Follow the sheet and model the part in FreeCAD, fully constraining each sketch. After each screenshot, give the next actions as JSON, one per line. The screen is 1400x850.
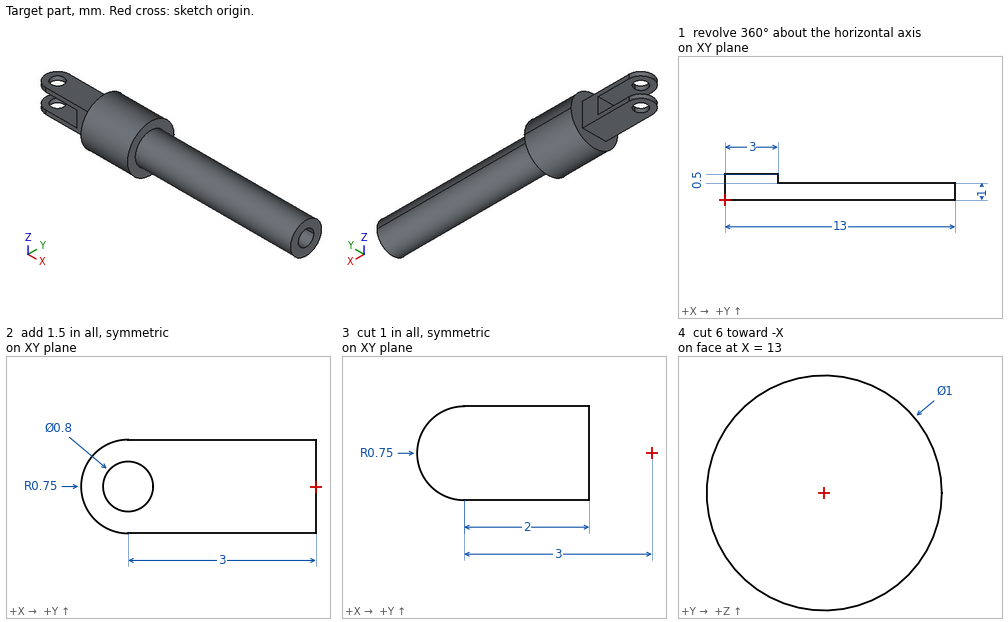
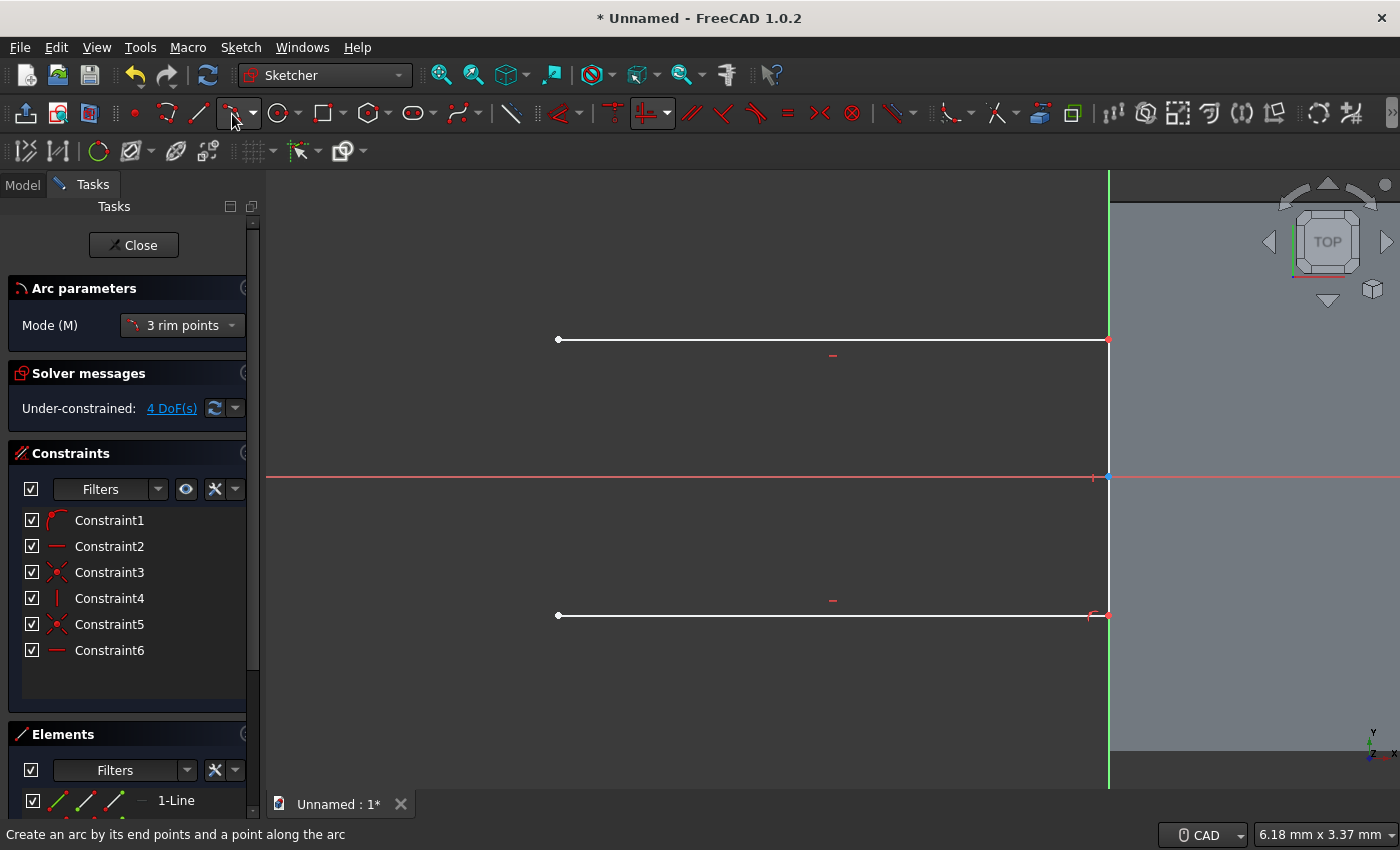
{"action": "left_click", "coordinate": [558, 340]}
{"action": "left_click", "coordinate": [558, 616]}
{"action": "left_click", "coordinate": [427, 434]}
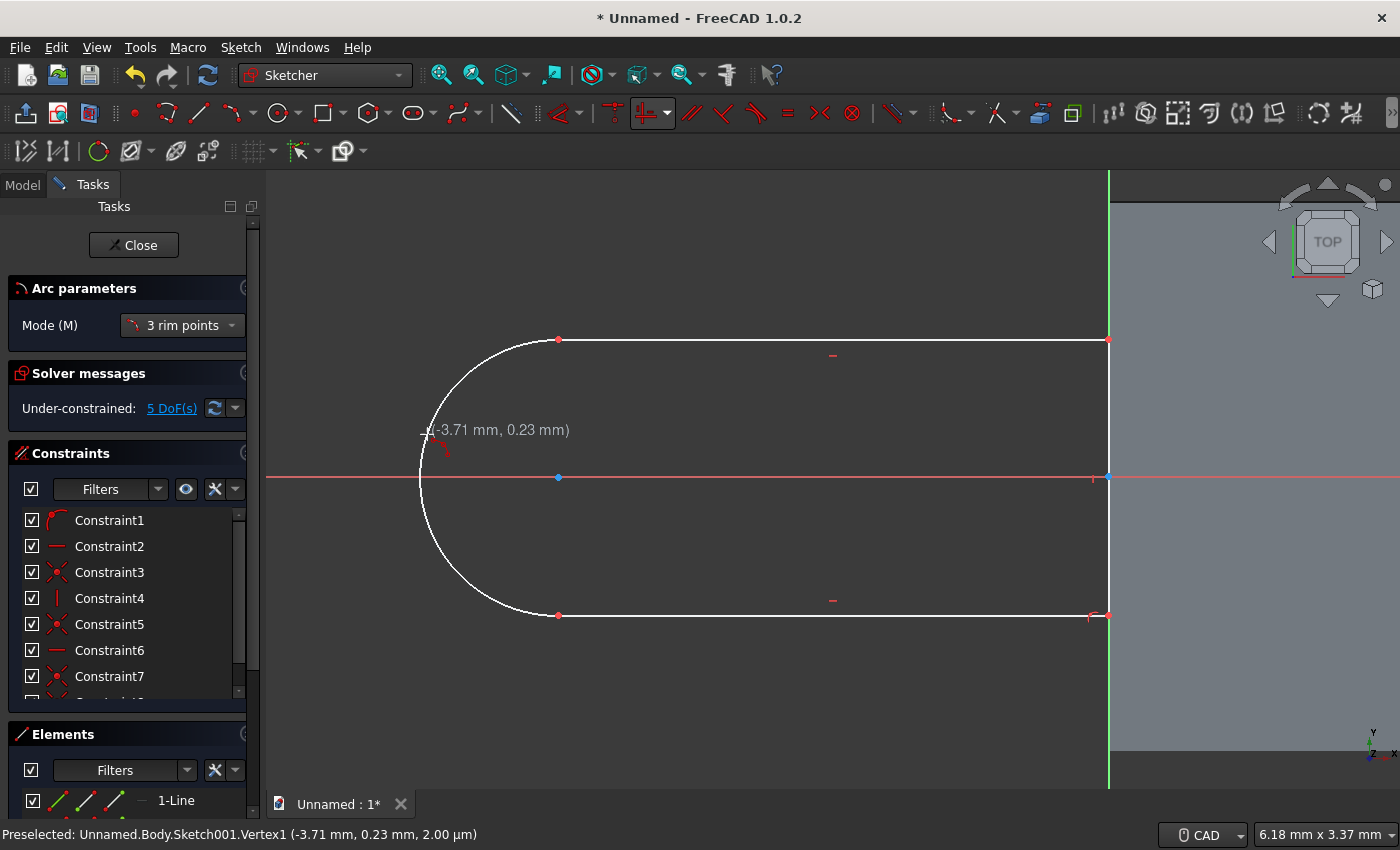
{"action": "left_click", "coordinate": [278, 114]}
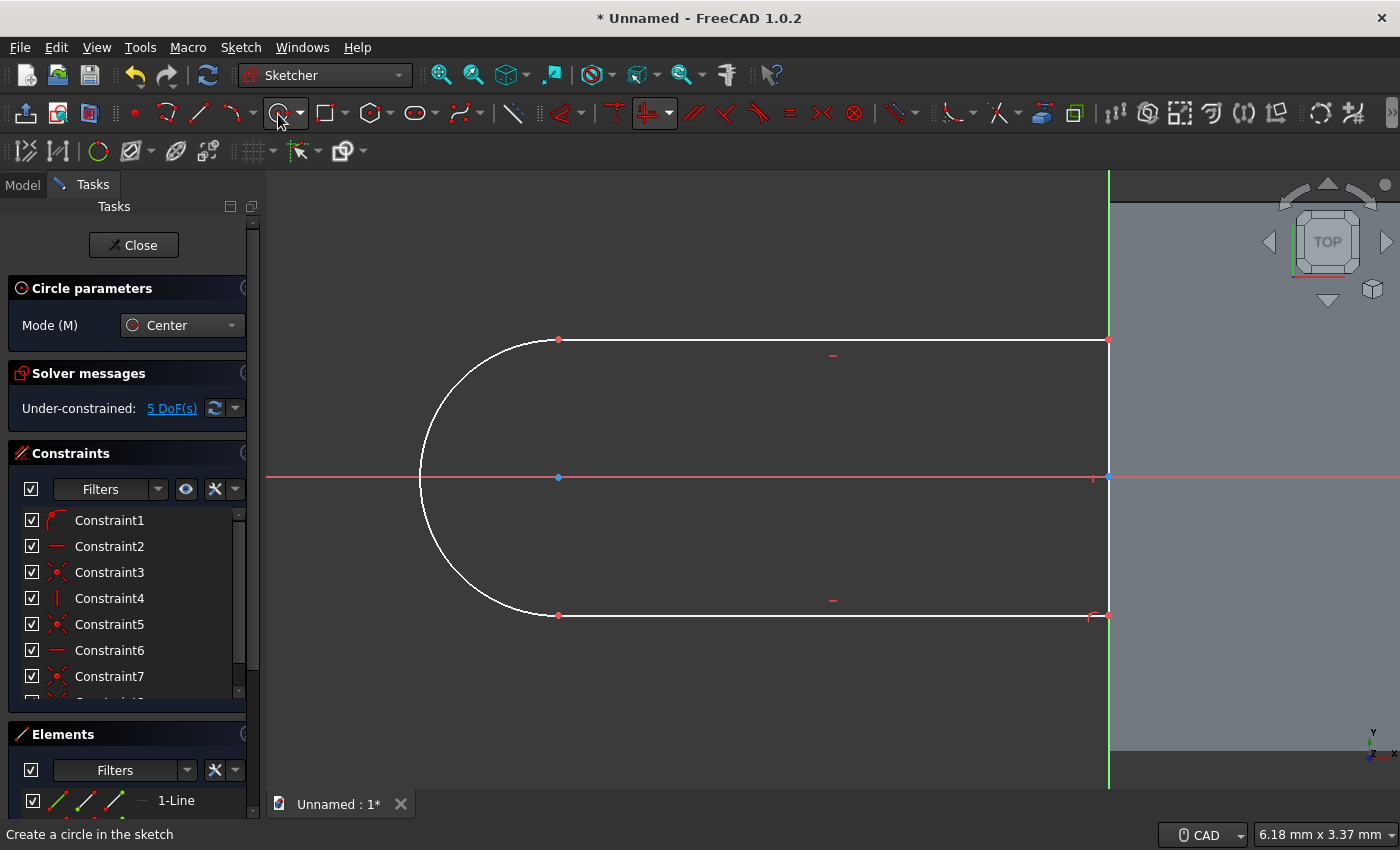
{"action": "left_click", "coordinate": [558, 477]}
{"action": "left_click", "coordinate": [610, 425]}
{"action": "key", "text": "Escape"}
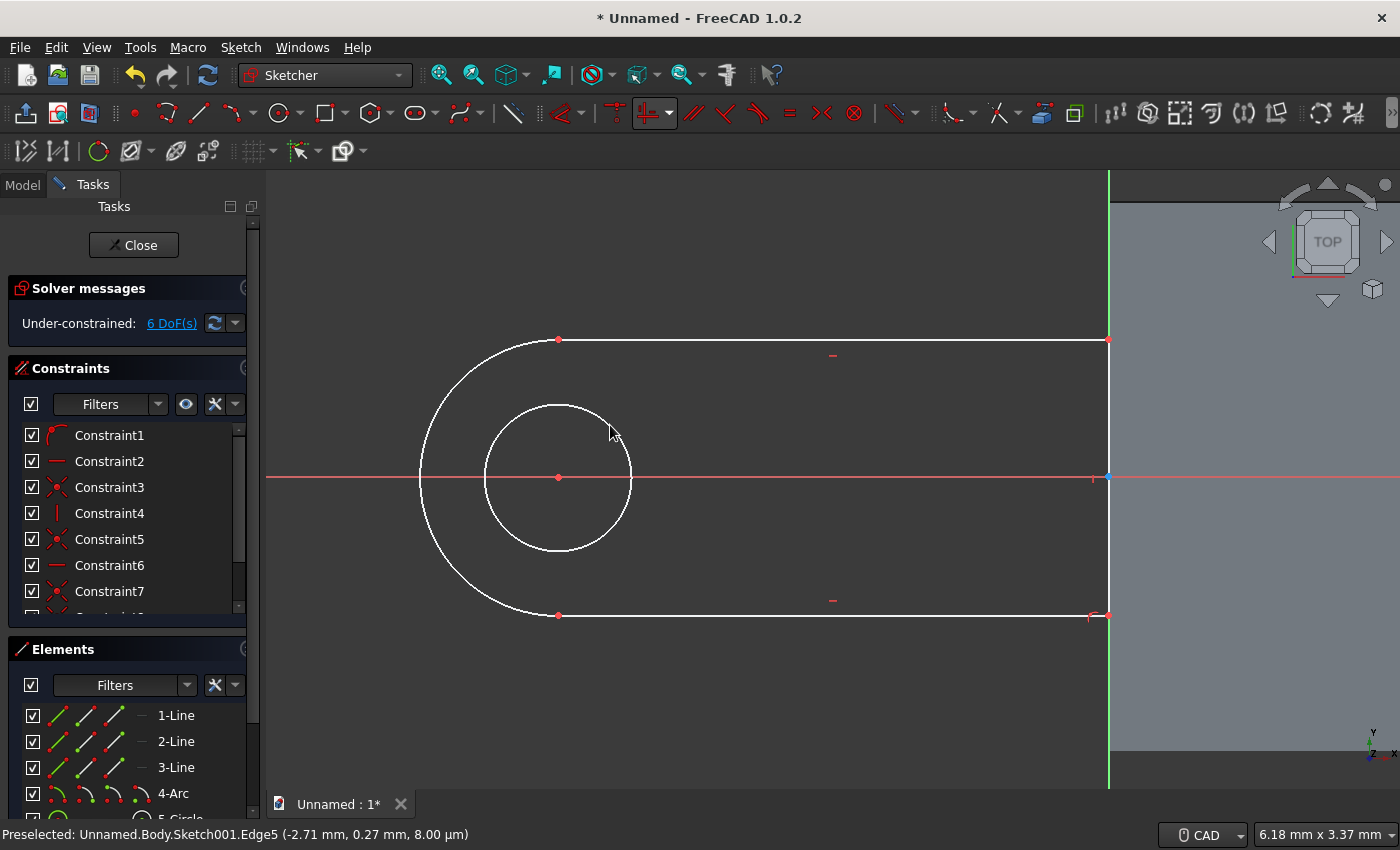
{"action": "left_click", "coordinate": [723, 616]}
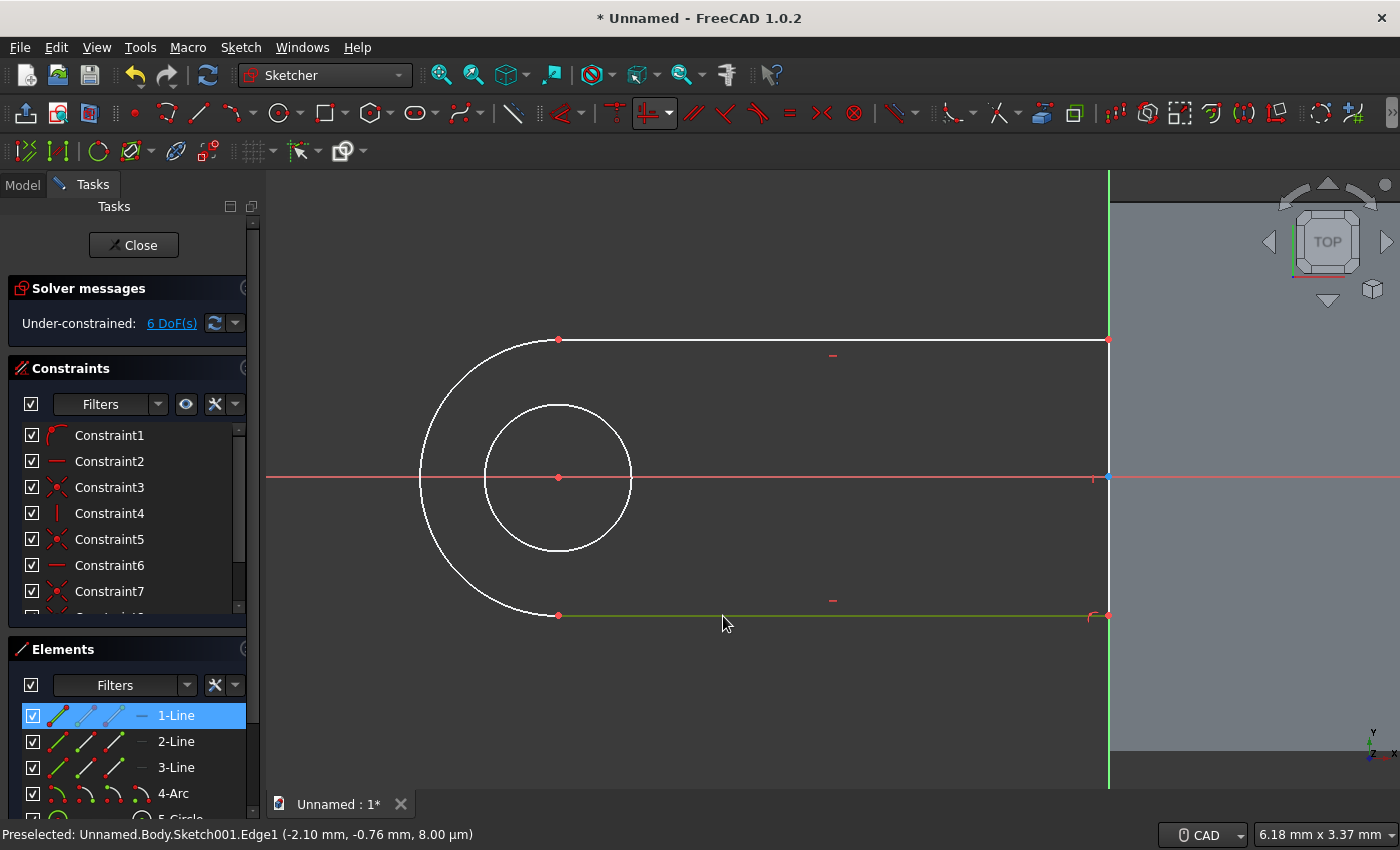
{"action": "left_click", "coordinate": [446, 397]}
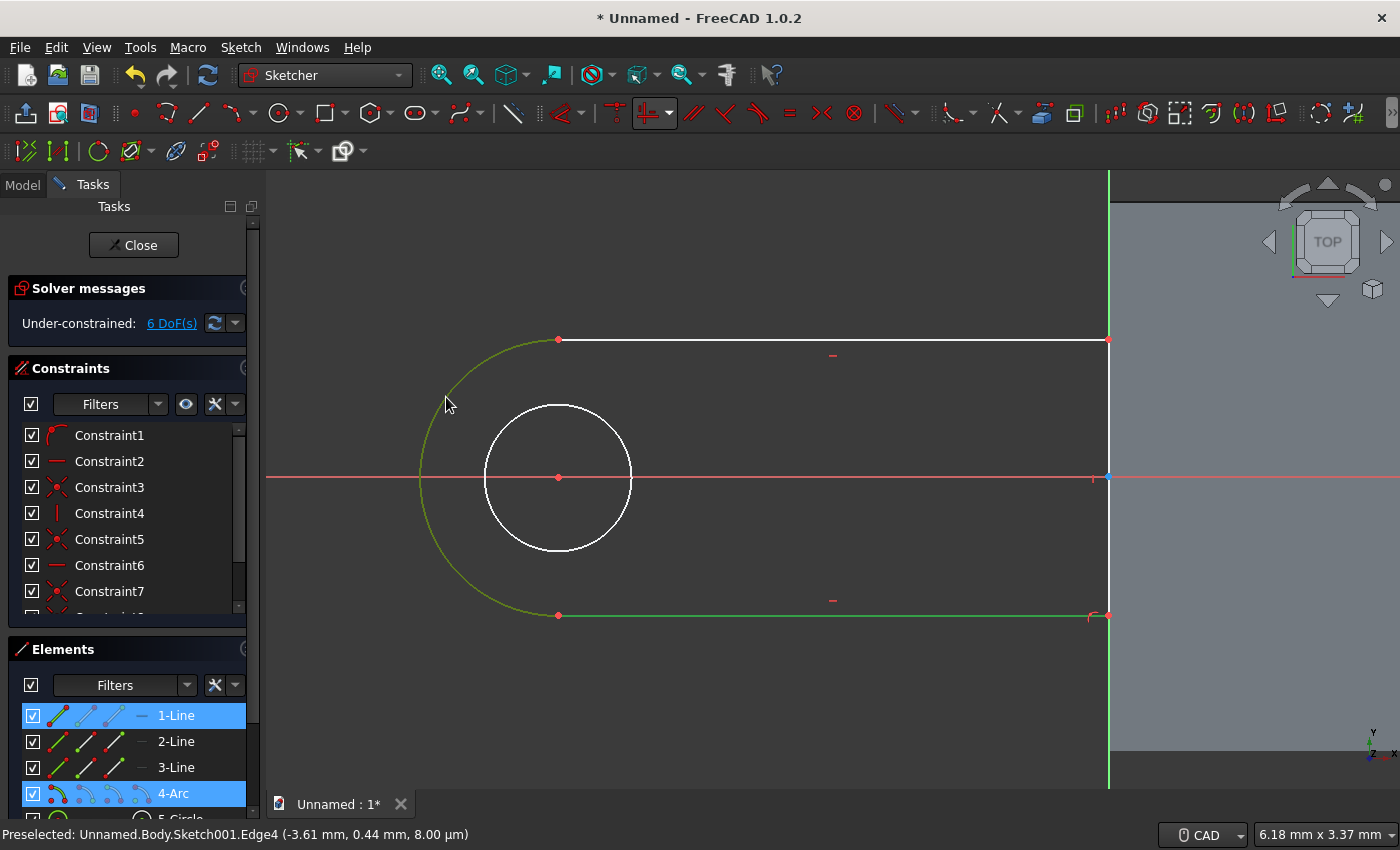
{"action": "key", "text": "t"}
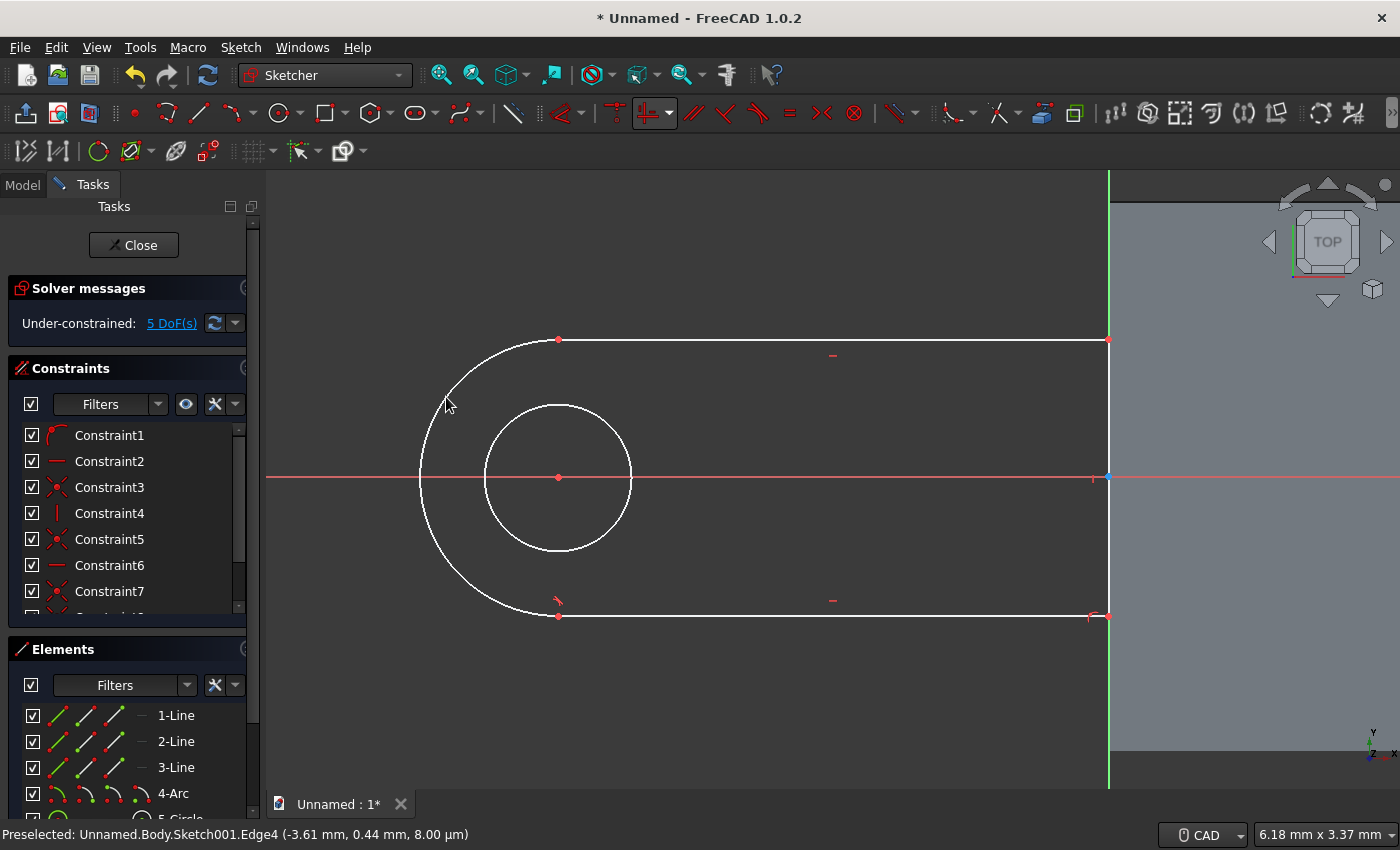
{"action": "left_click", "coordinate": [944, 340]}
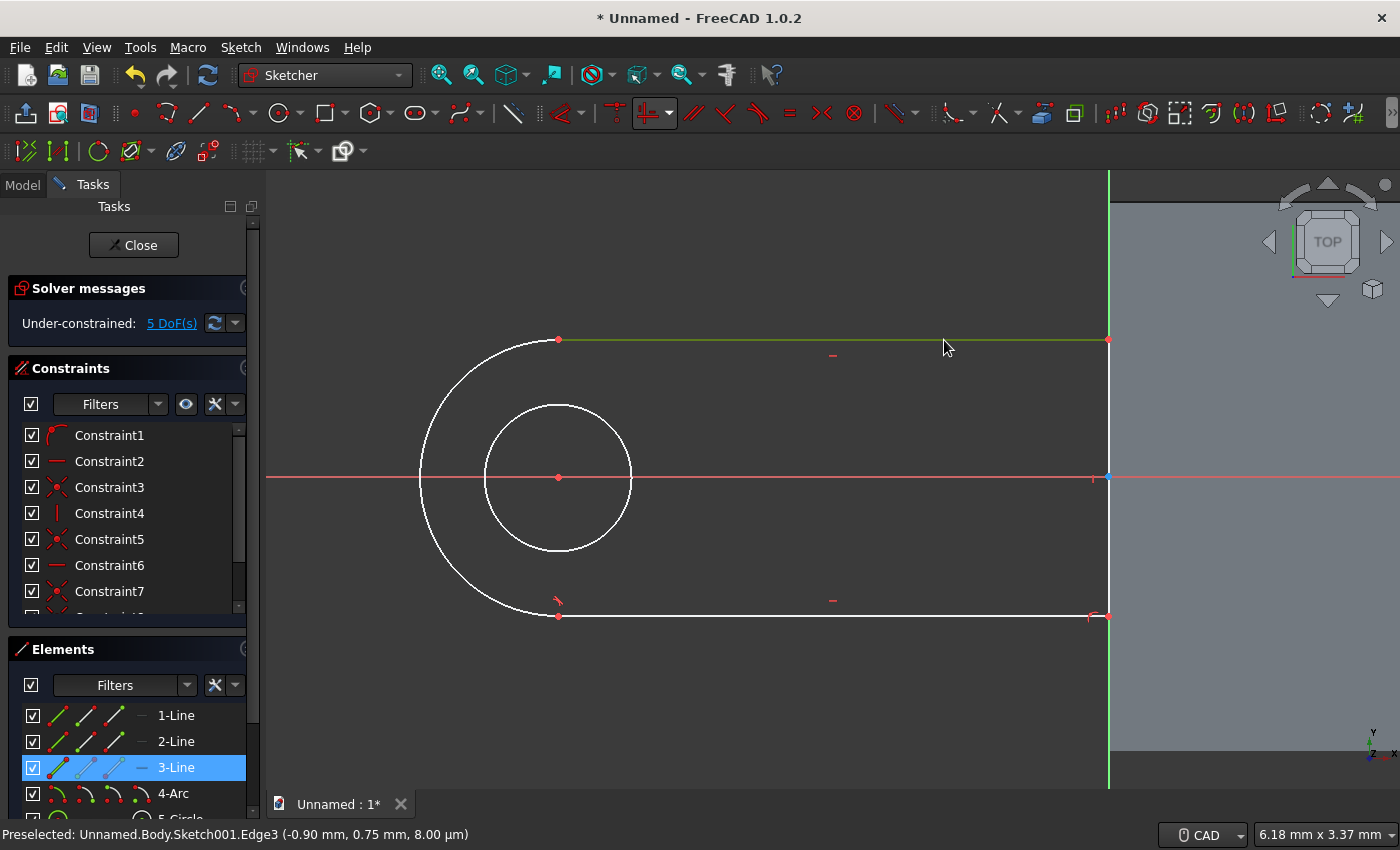
{"action": "left_click", "coordinate": [446, 397]}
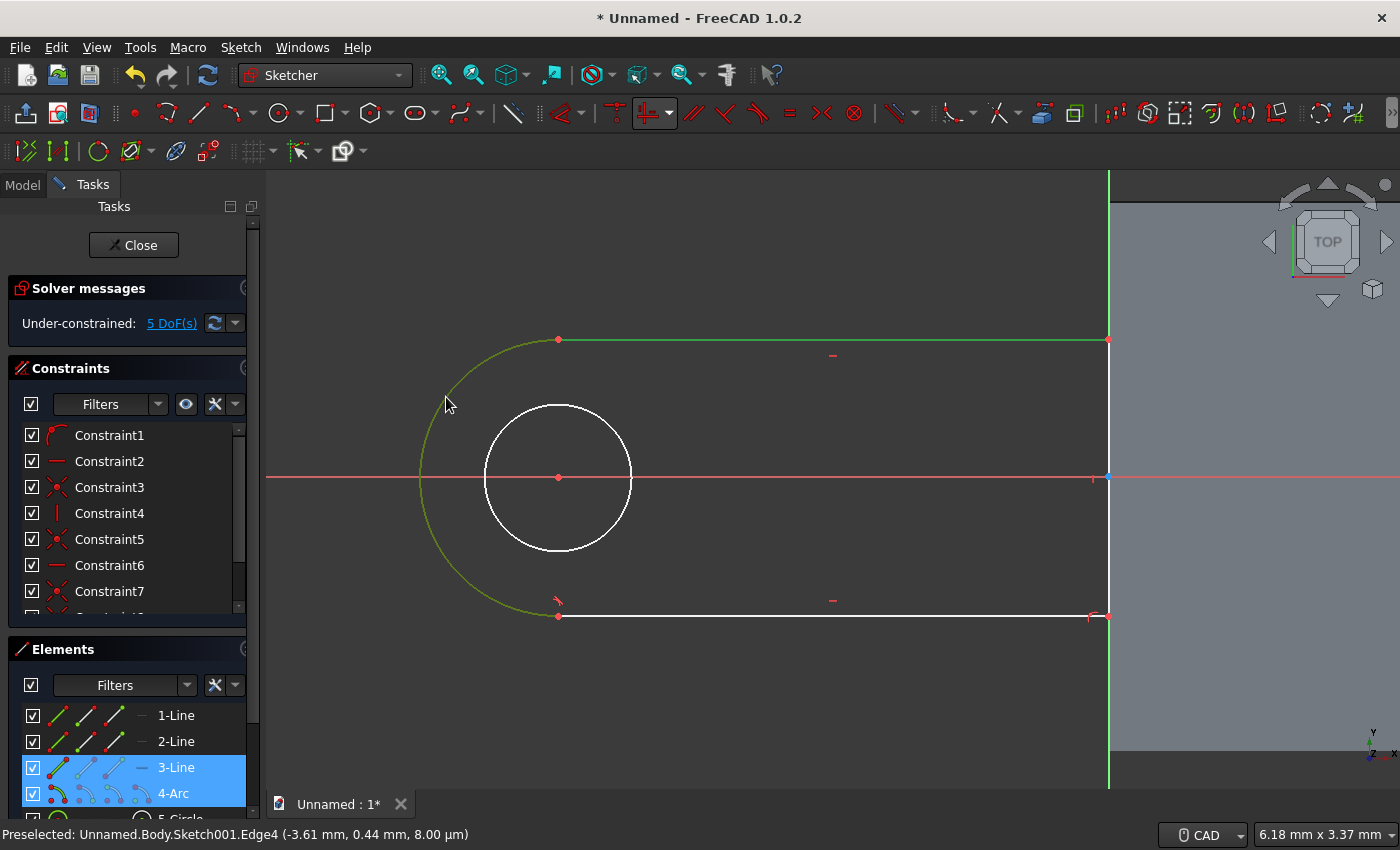
{"action": "left_click", "coordinate": [758, 114]}